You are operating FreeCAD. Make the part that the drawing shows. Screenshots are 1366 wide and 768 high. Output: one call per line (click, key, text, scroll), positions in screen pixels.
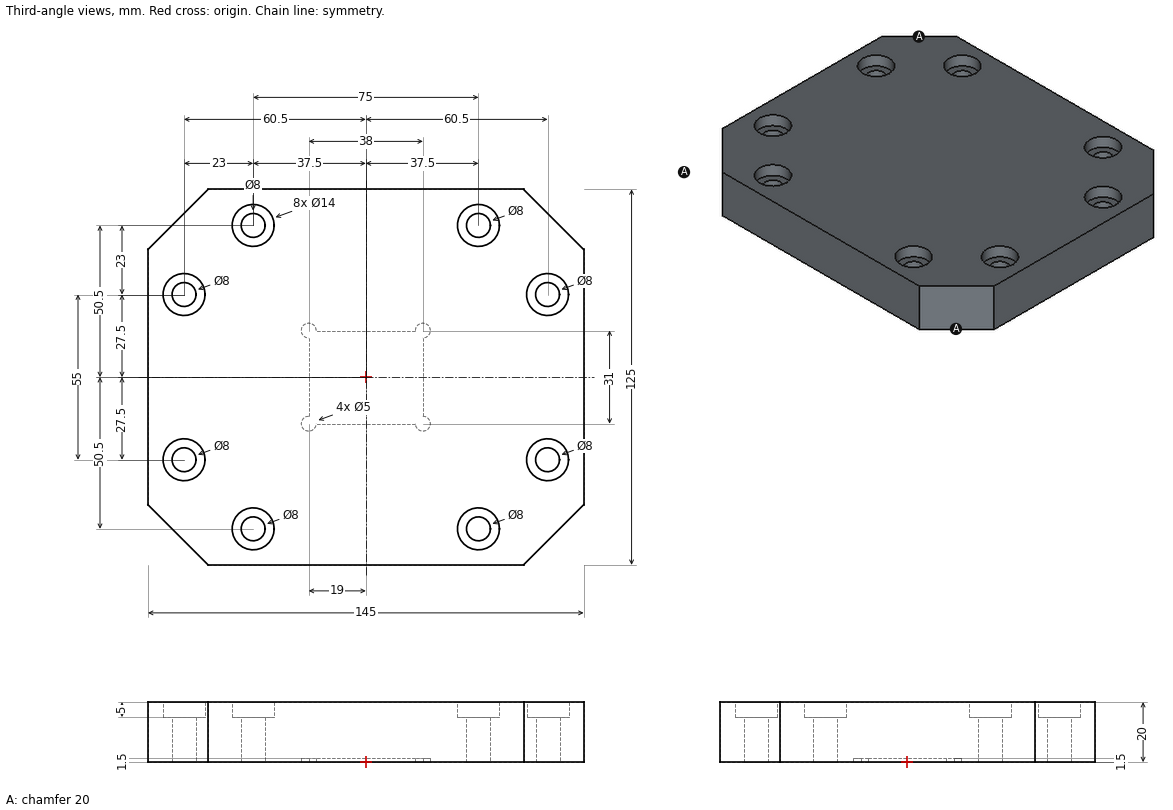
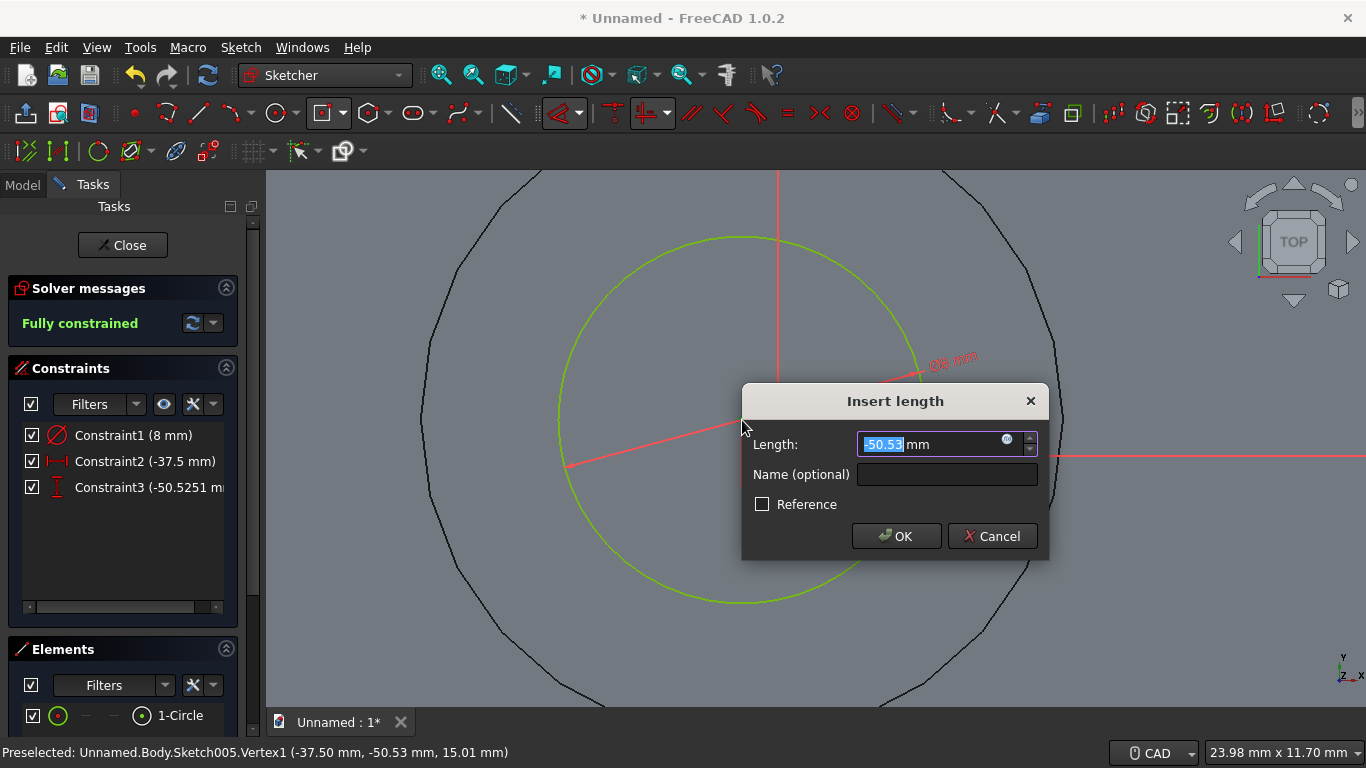
text(-50.5)
key(Return)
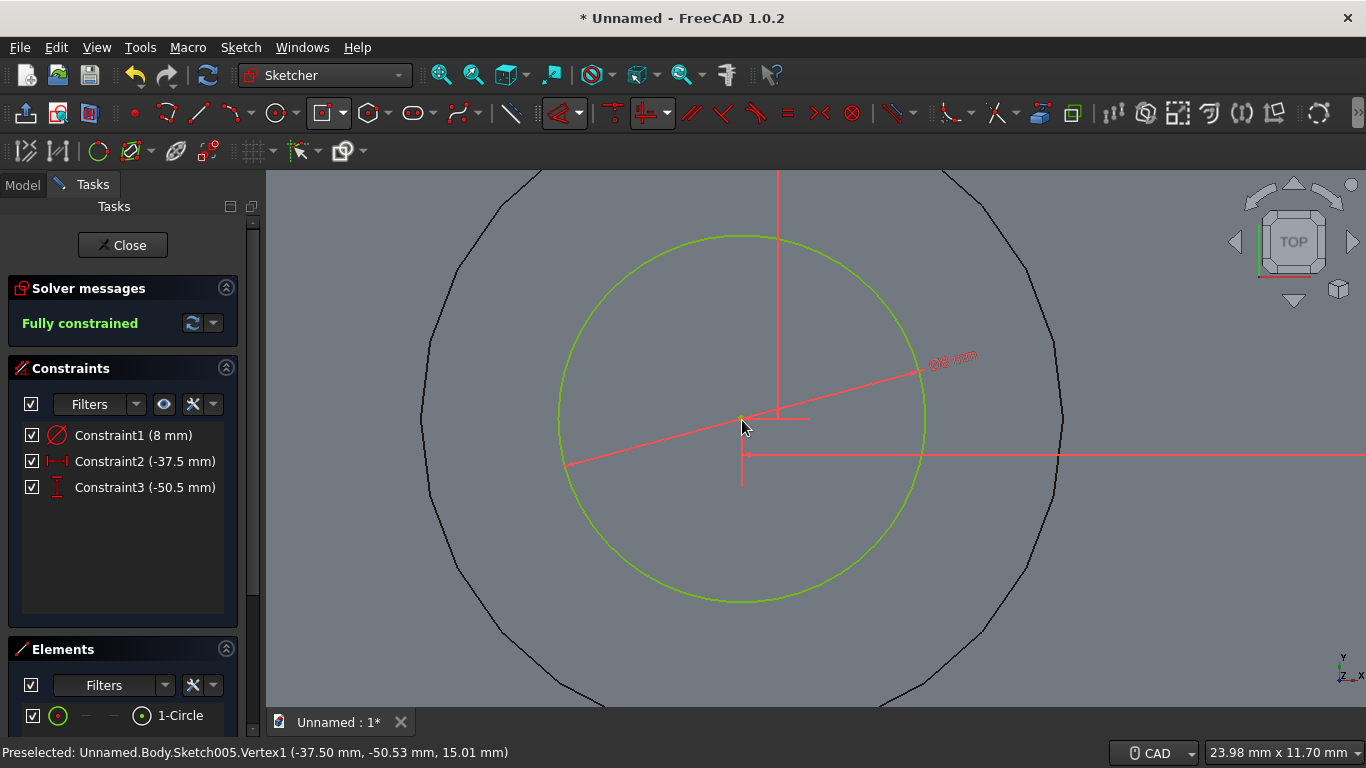
click(123, 245)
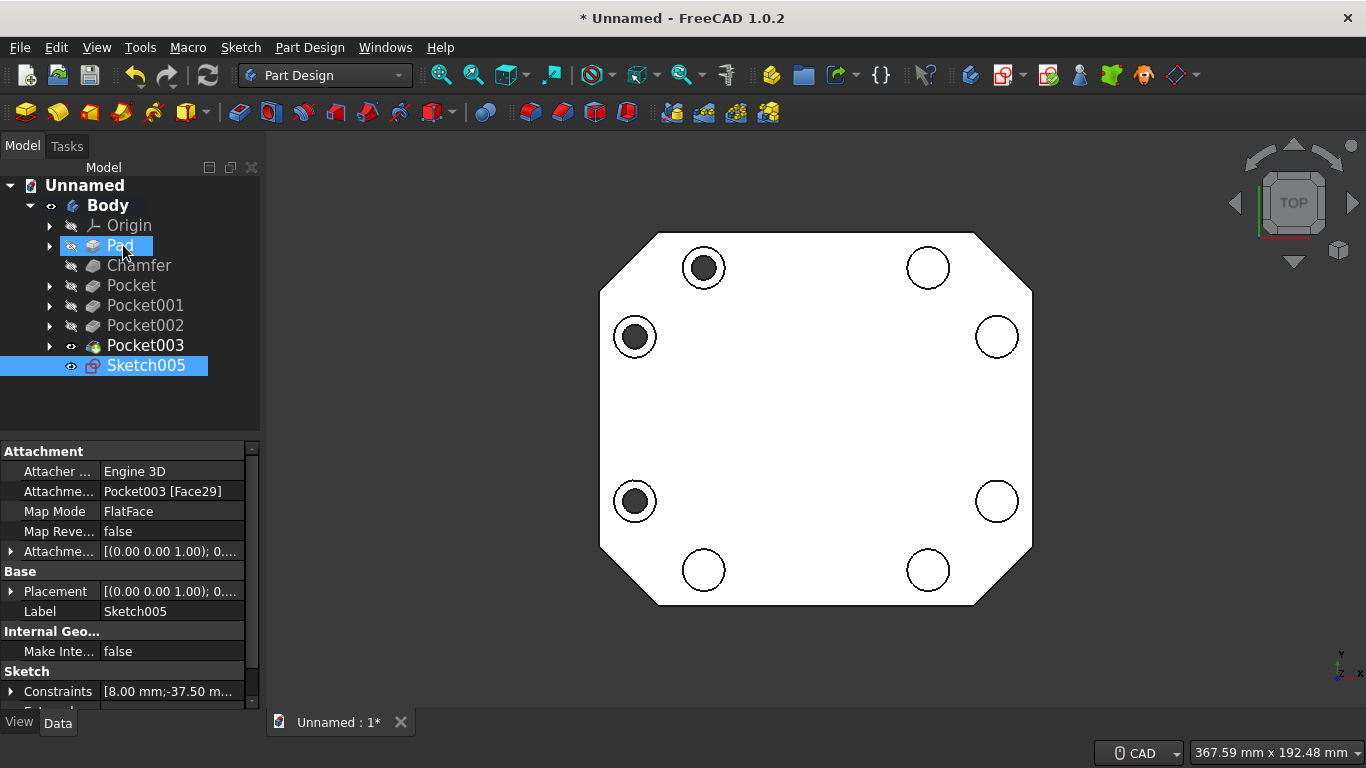
click(240, 112)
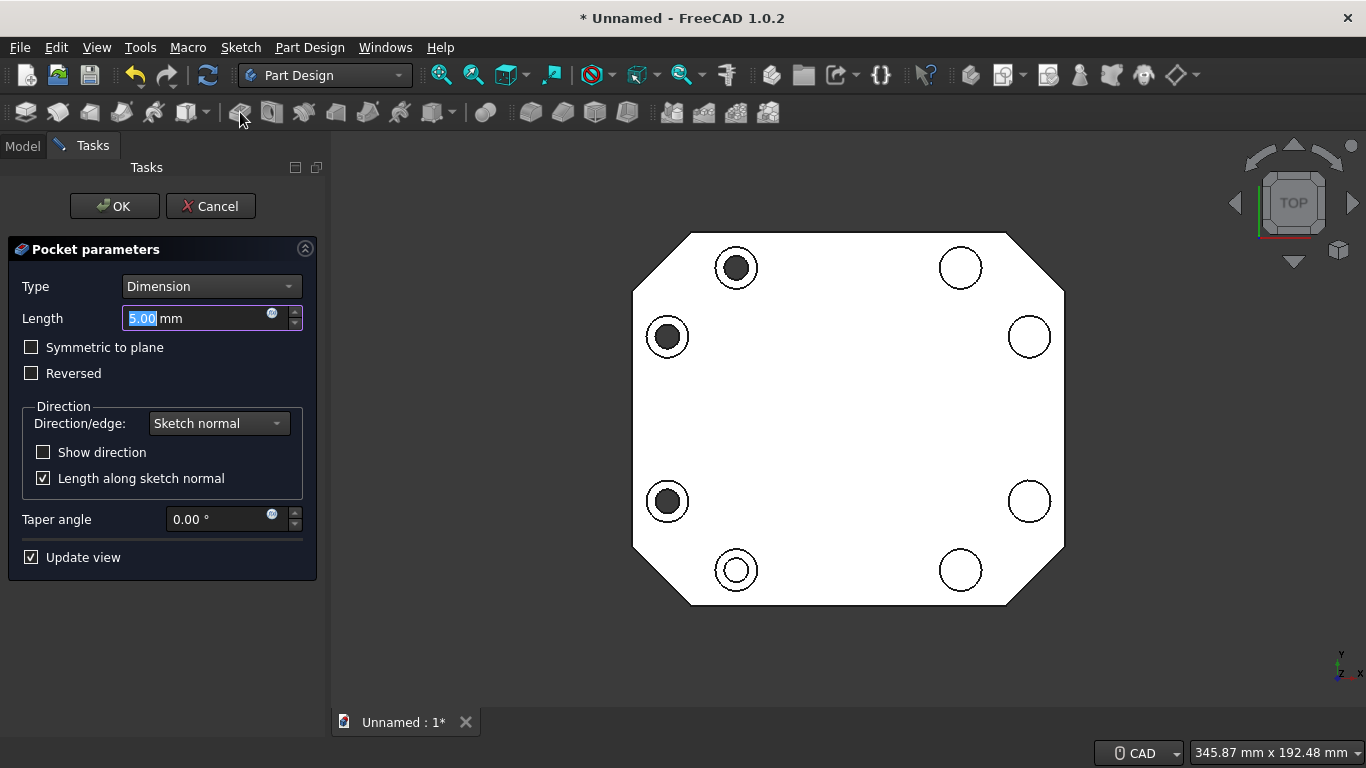
click(212, 286)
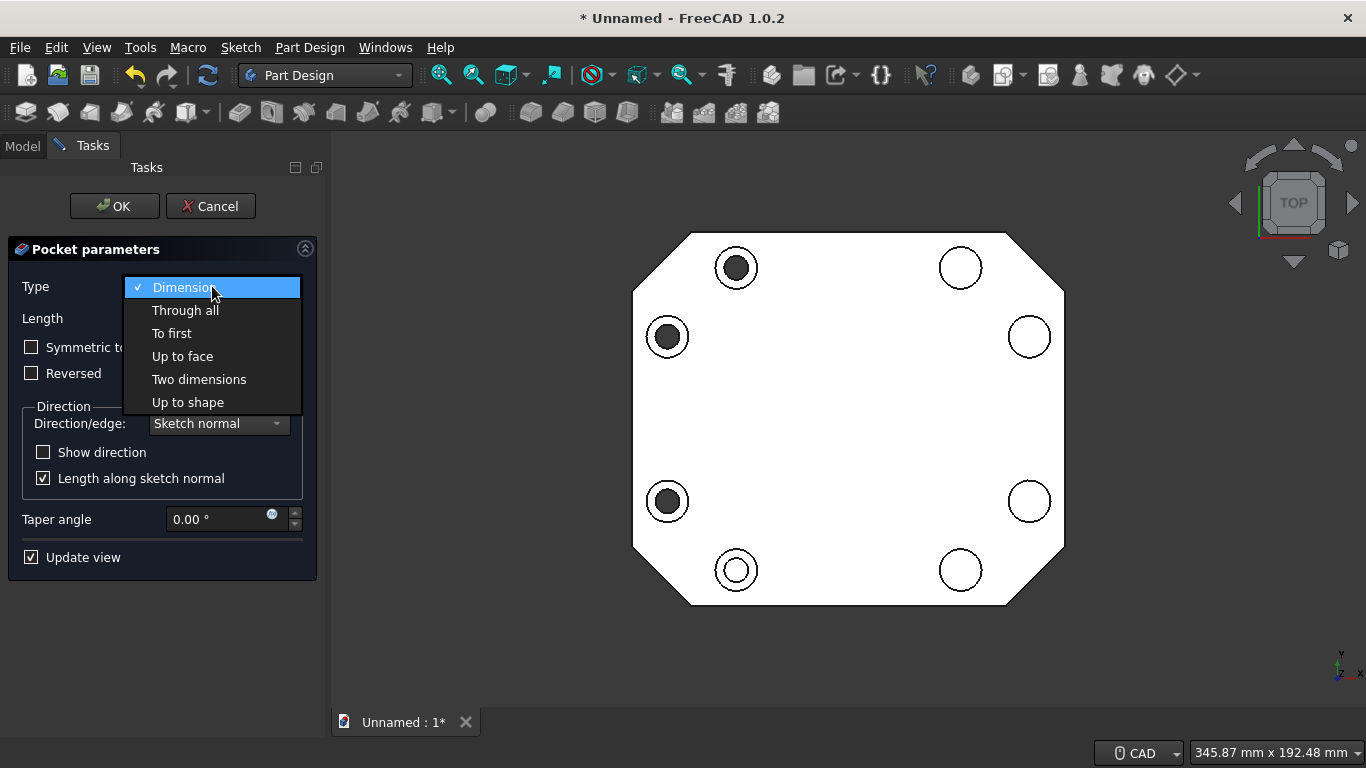
click(212, 334)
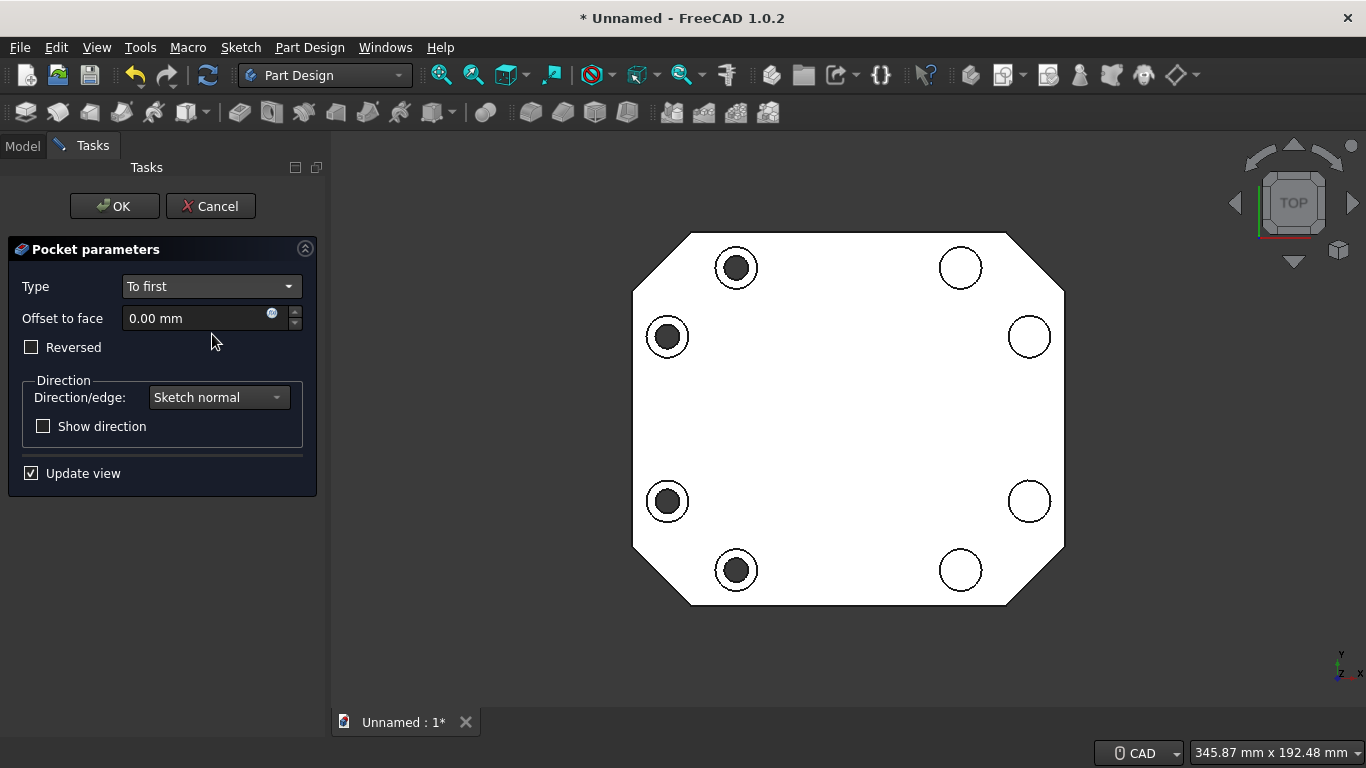
click(115, 206)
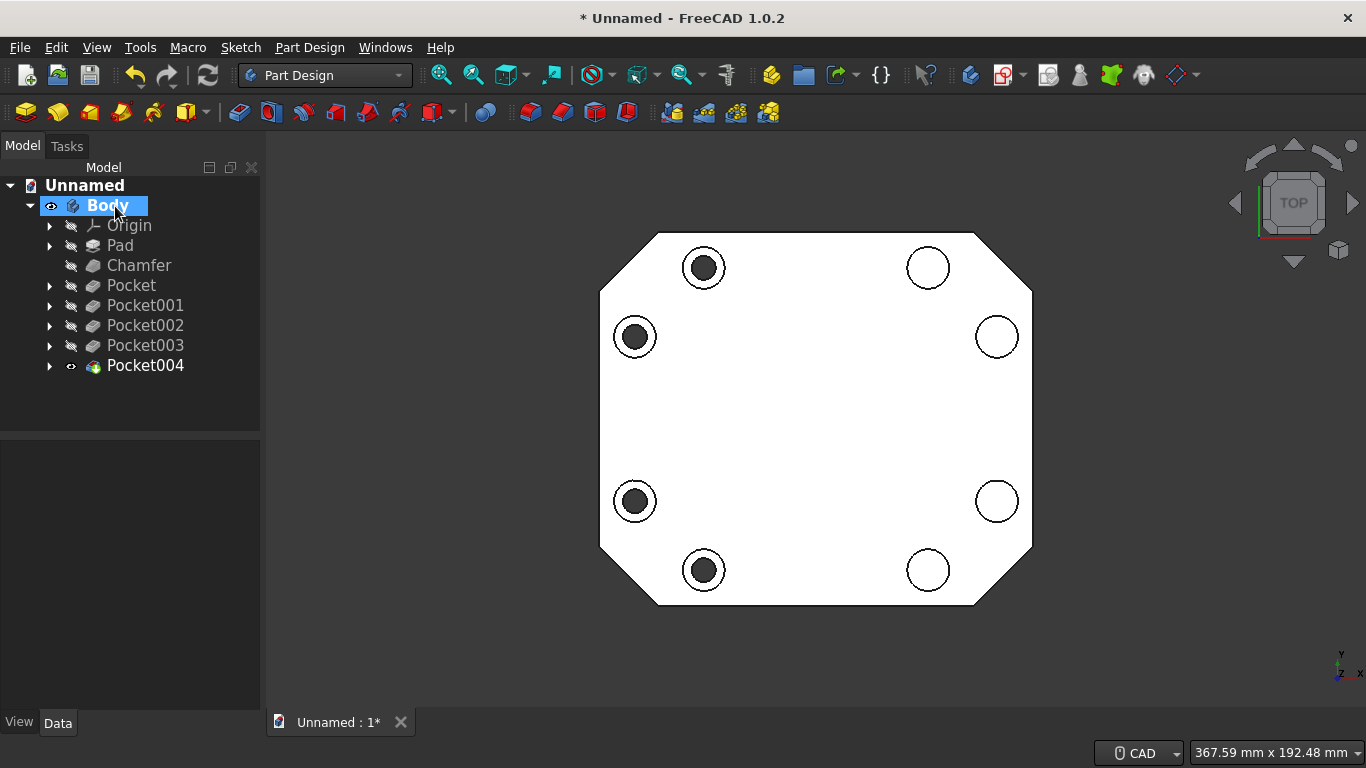
click(928, 267)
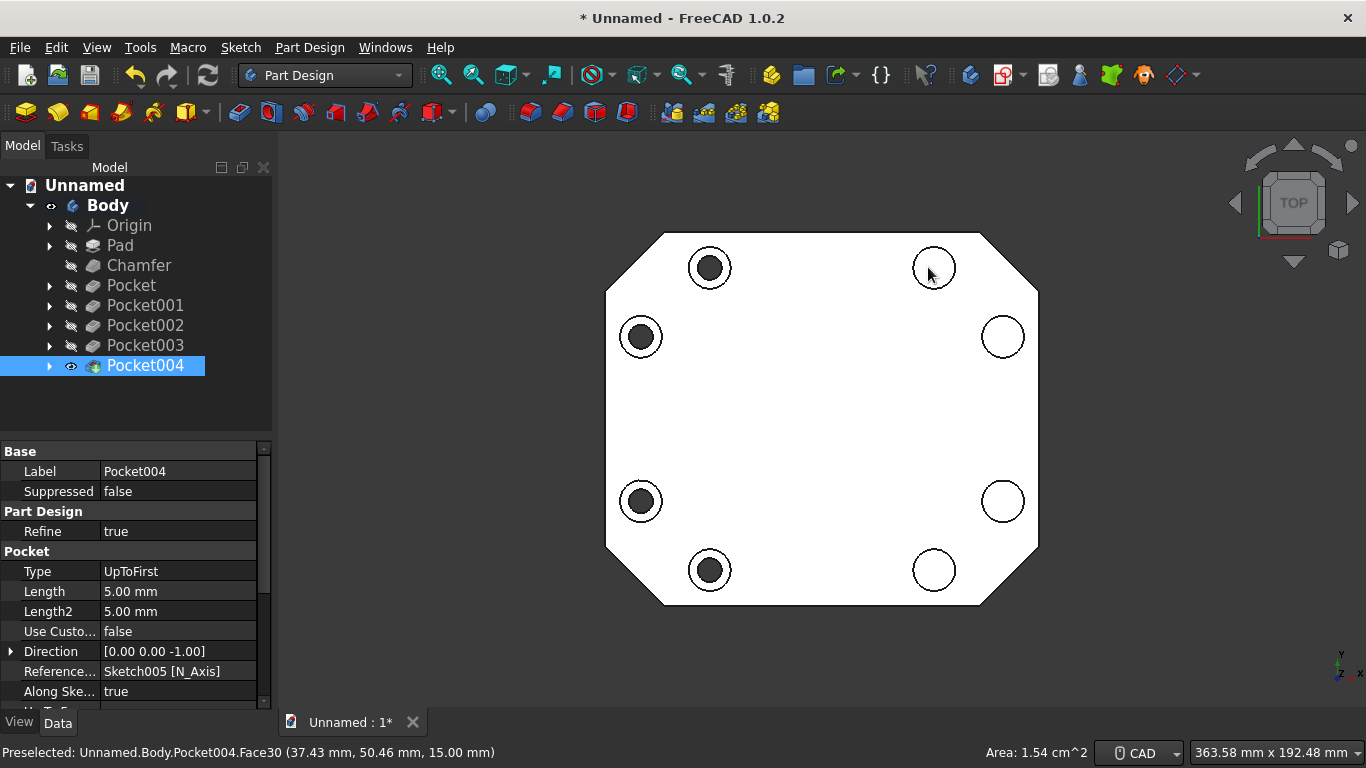
click(1004, 76)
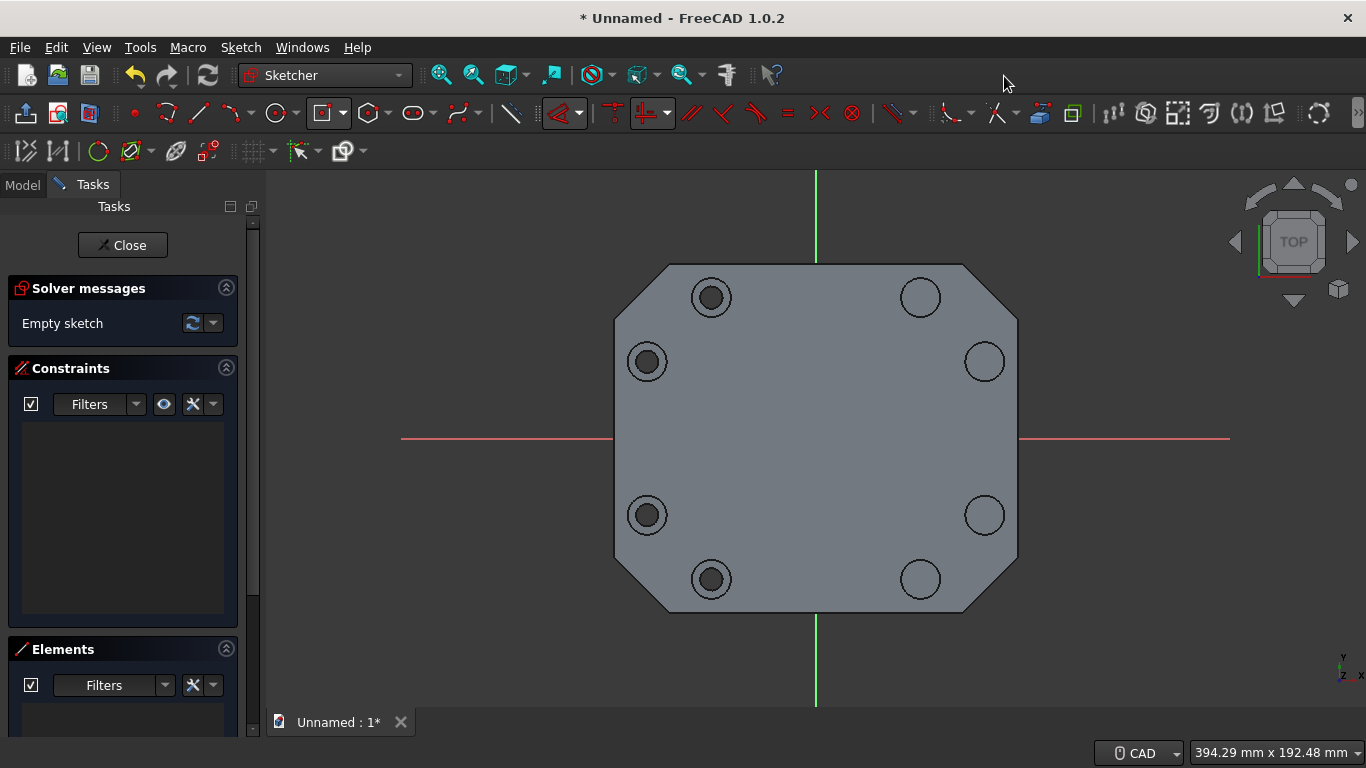
key(q)
key(s)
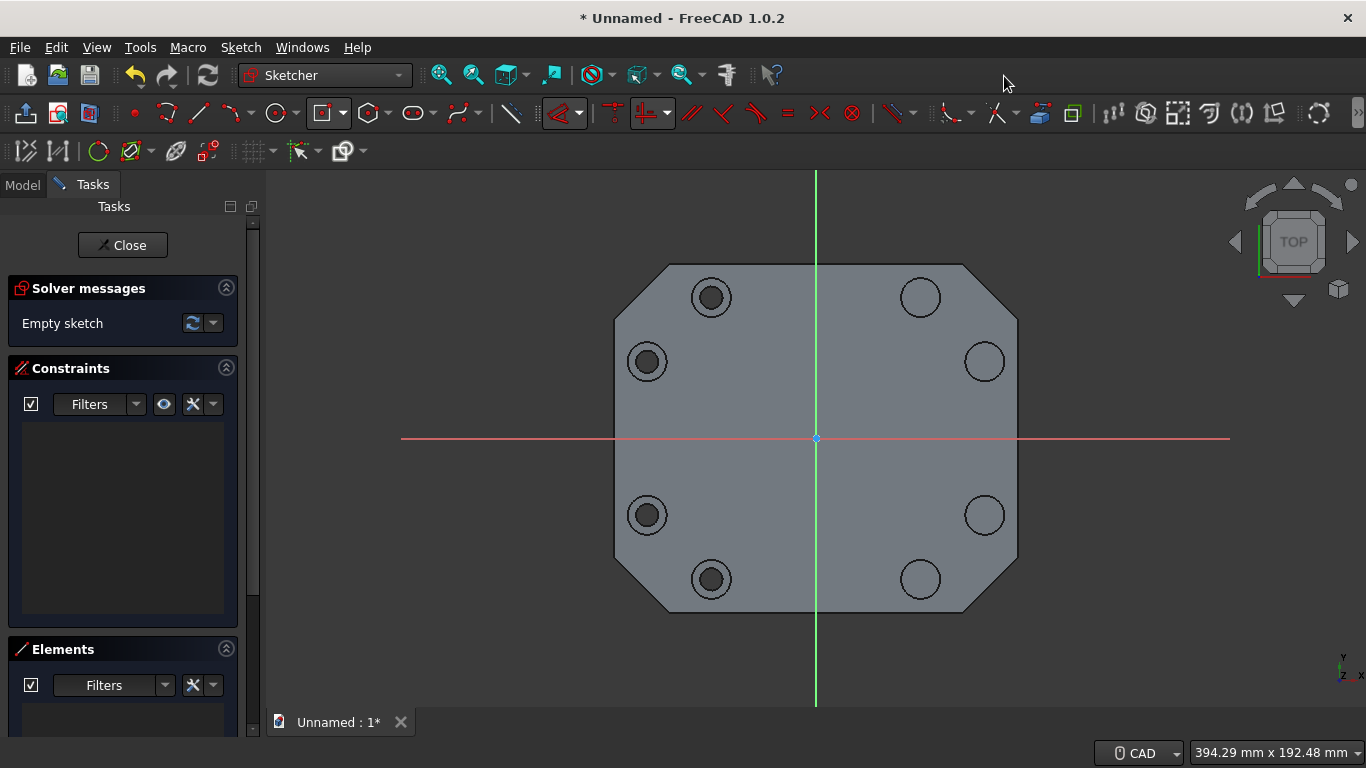
scroll(932, 288, up, 14)